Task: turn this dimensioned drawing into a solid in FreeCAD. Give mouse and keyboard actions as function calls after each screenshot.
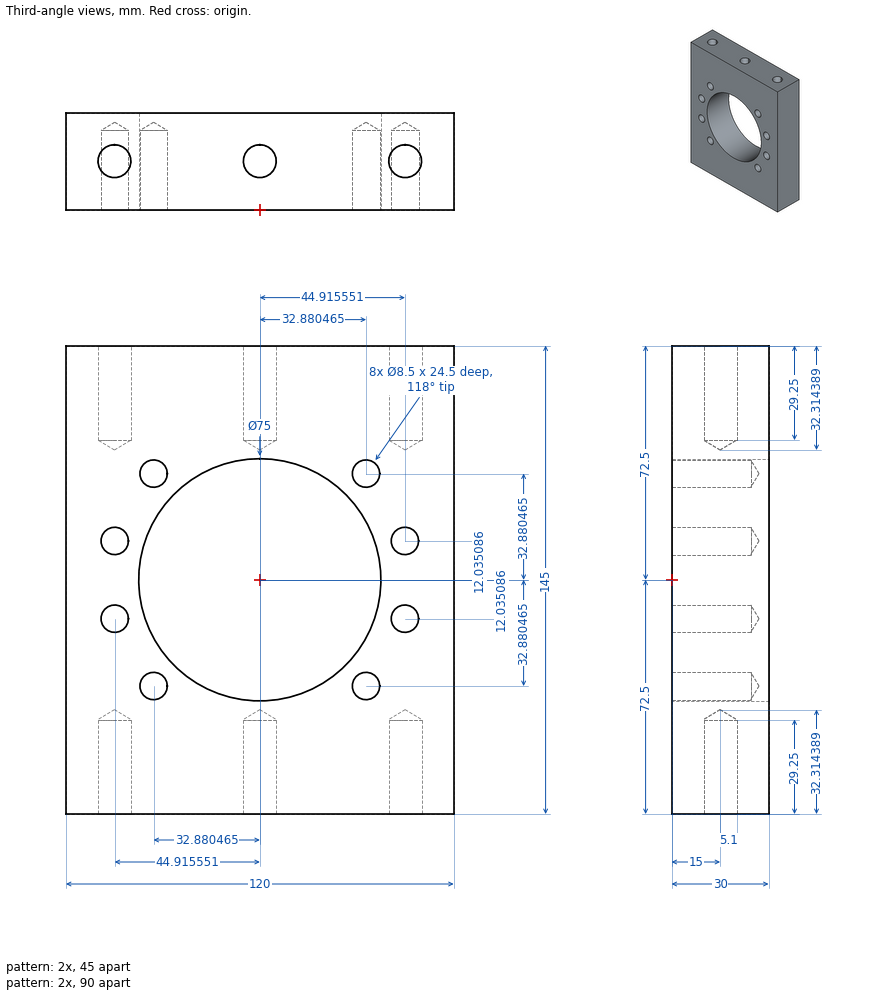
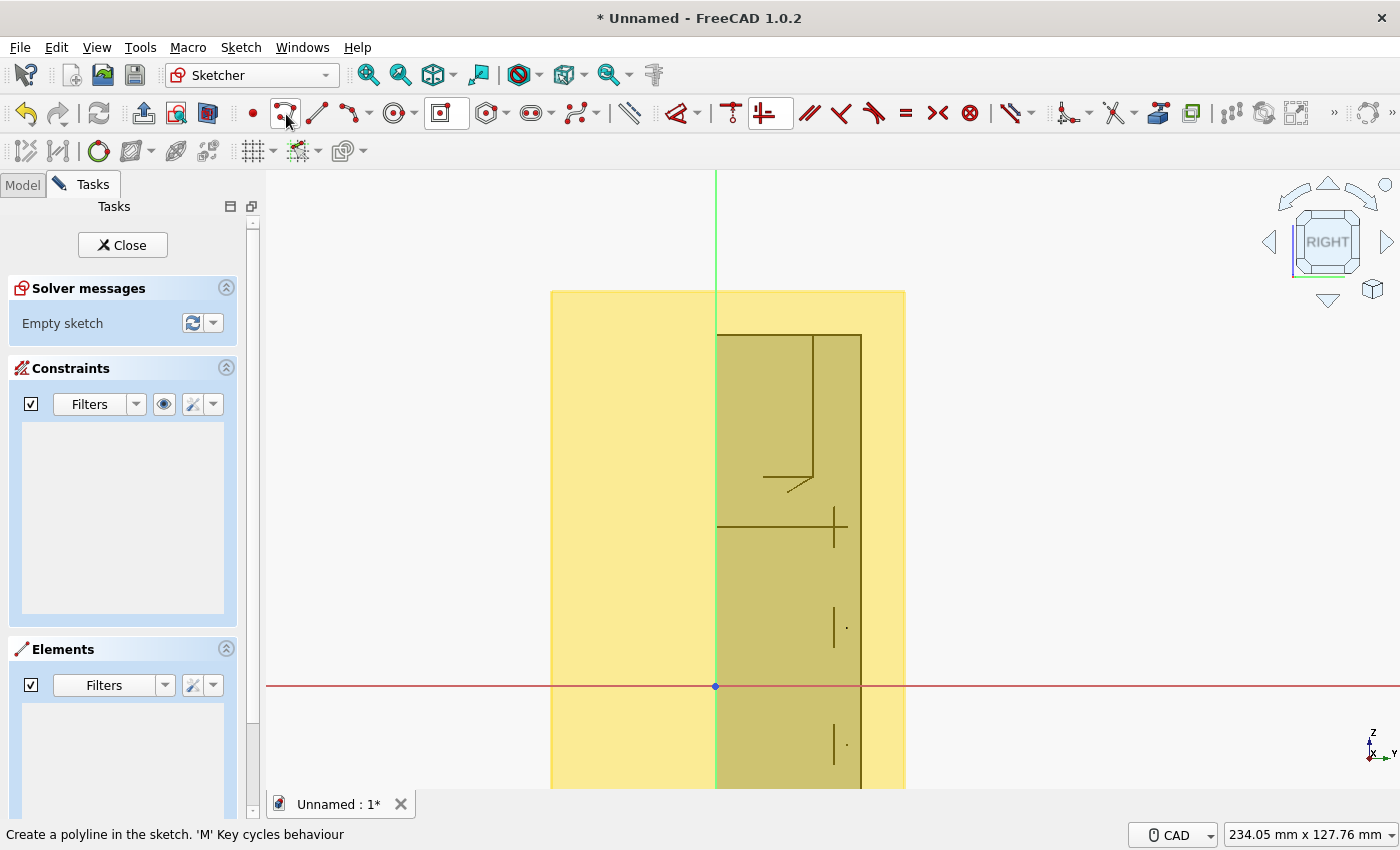
click(788, 492)
click(813, 477)
click(813, 335)
click(788, 335)
click(788, 493)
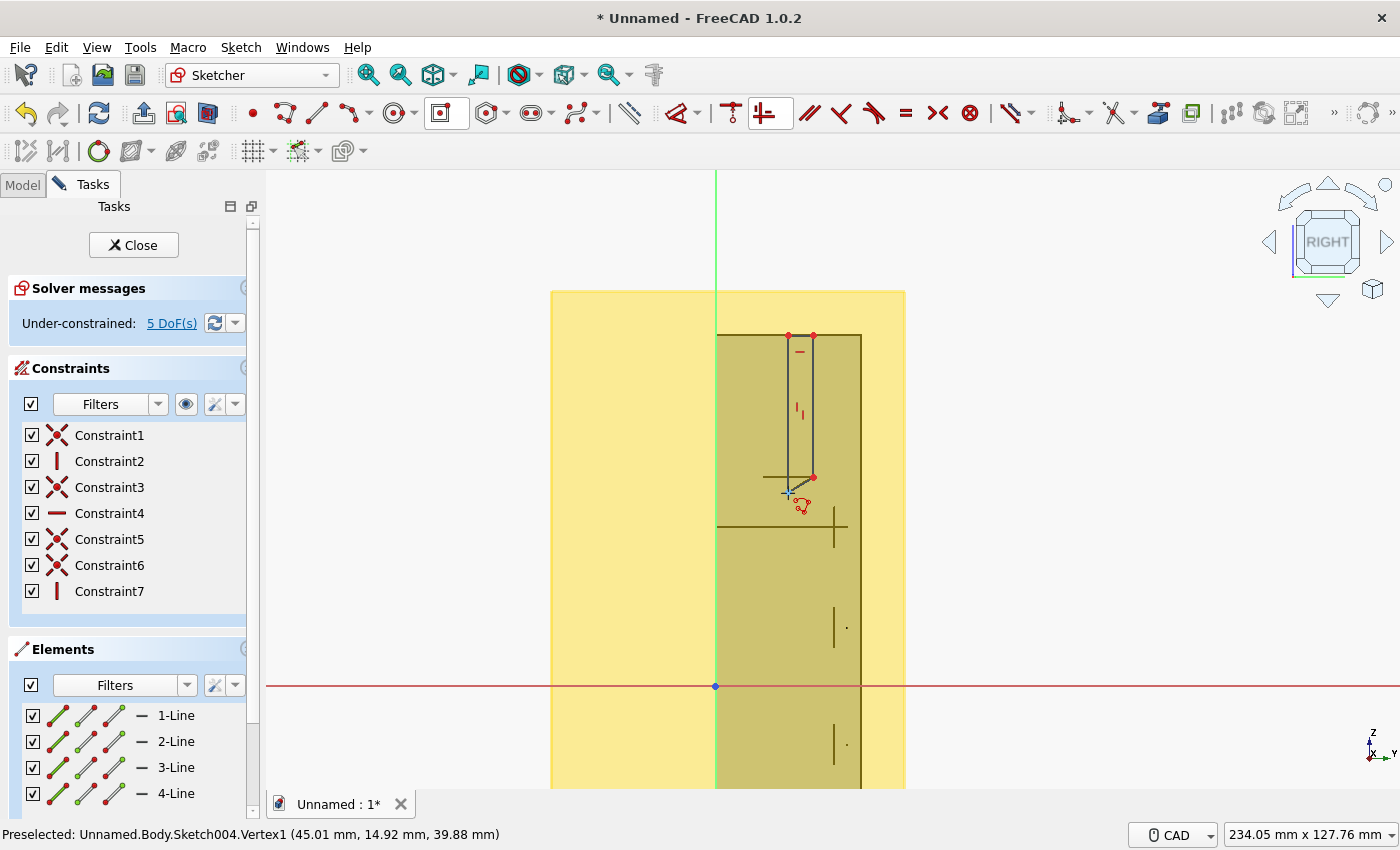
click(318, 114)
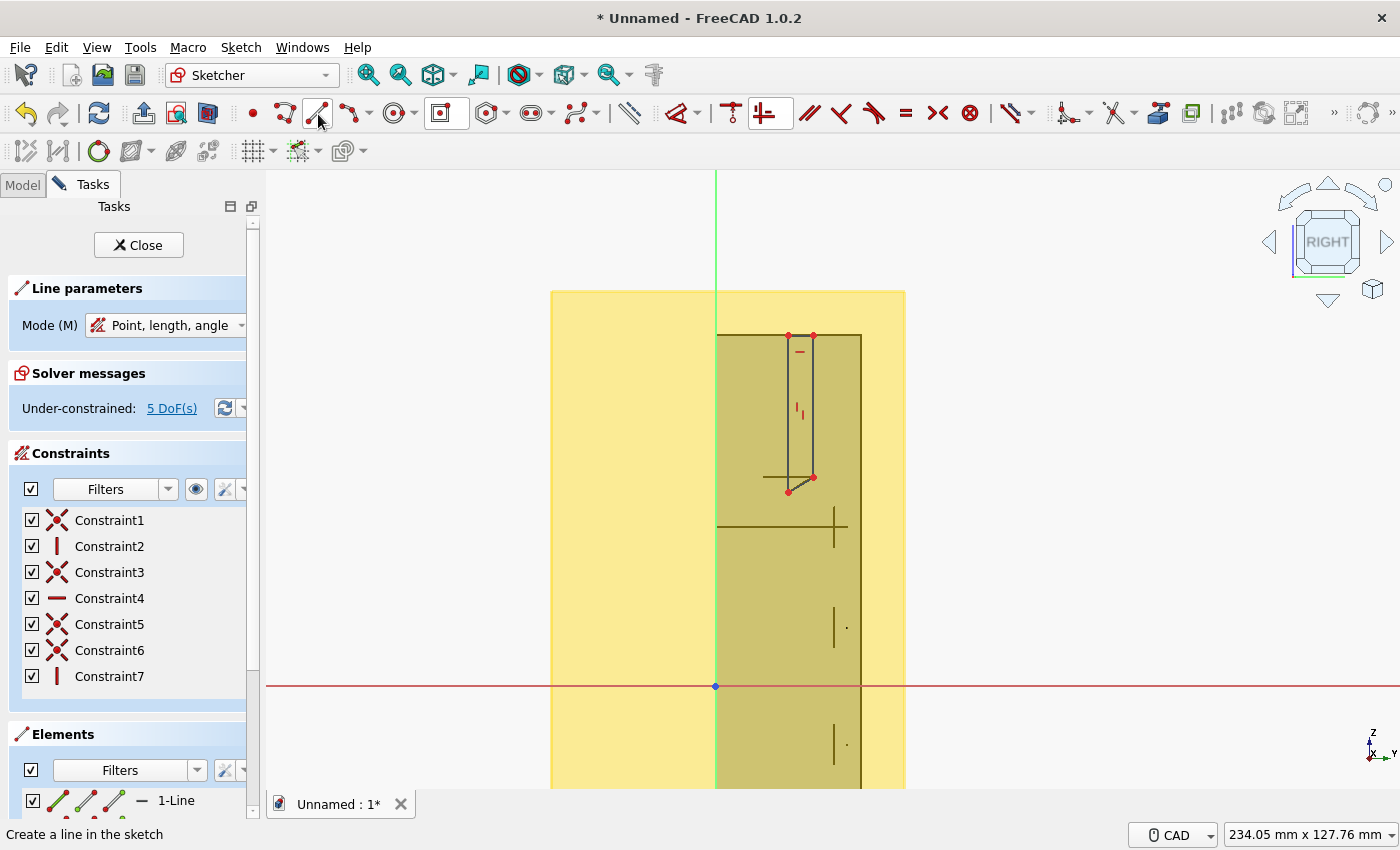
click(788, 319)
click(788, 272)
key(Escape)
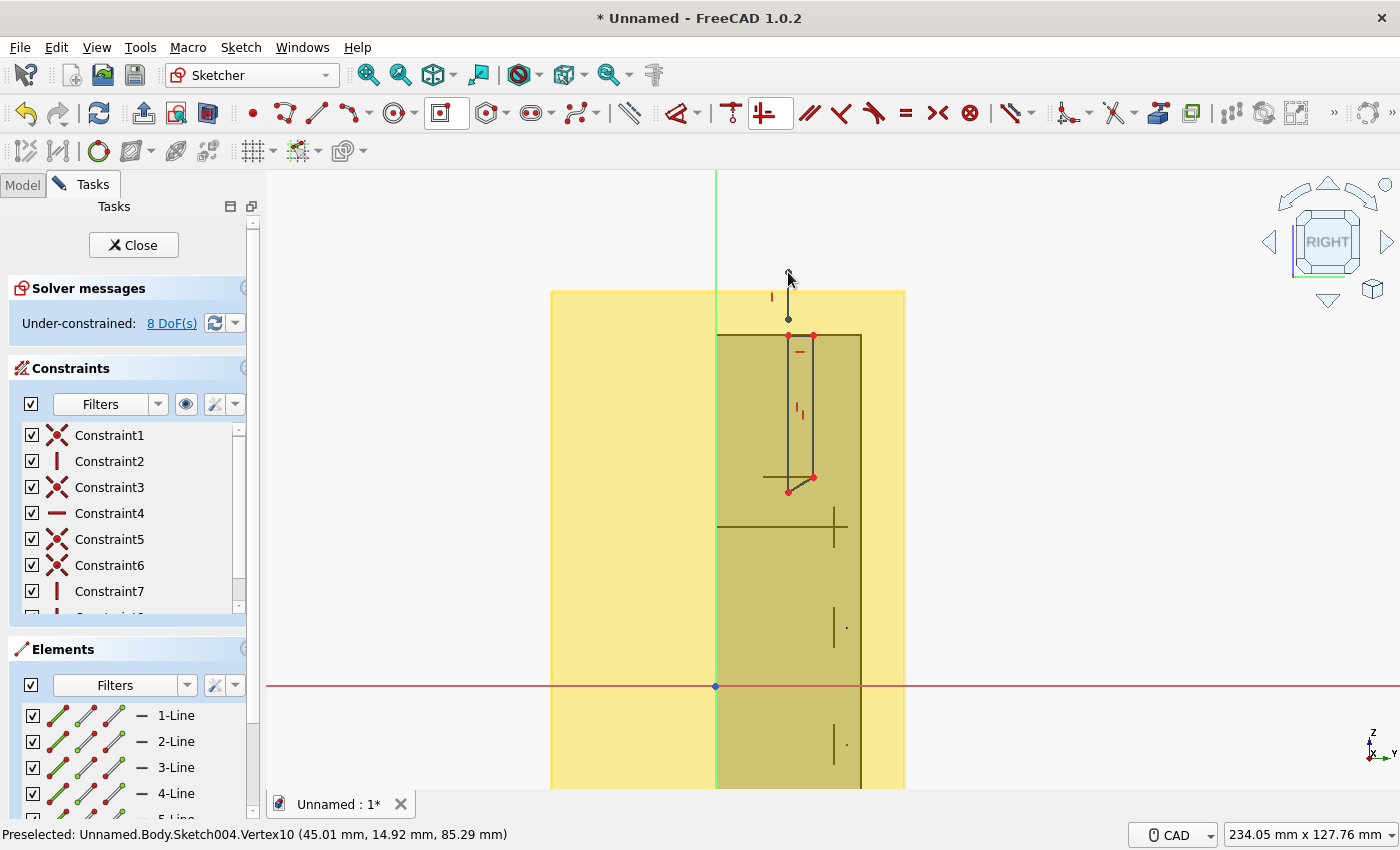
click(788, 306)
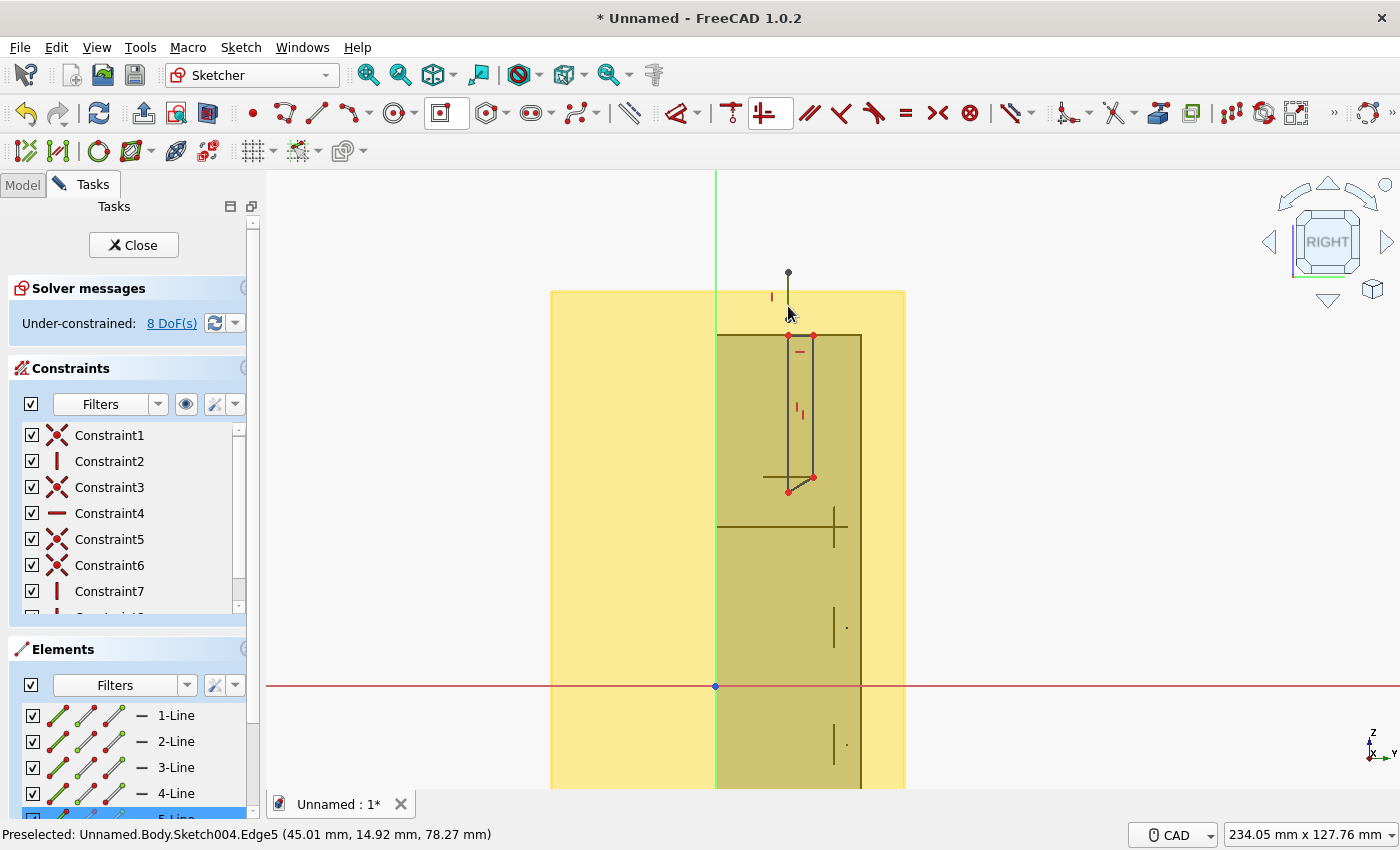
click(630, 114)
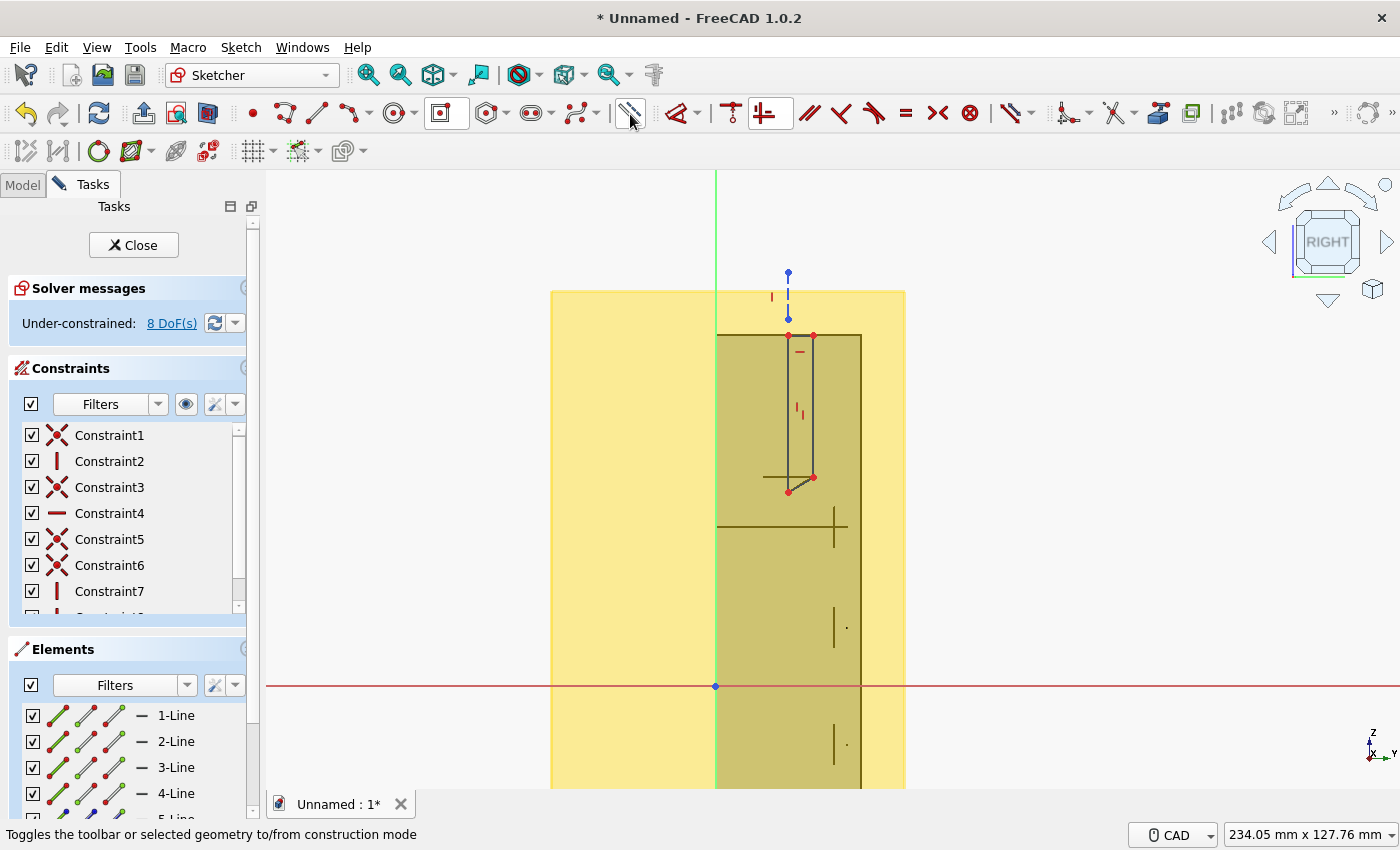
click(676, 114)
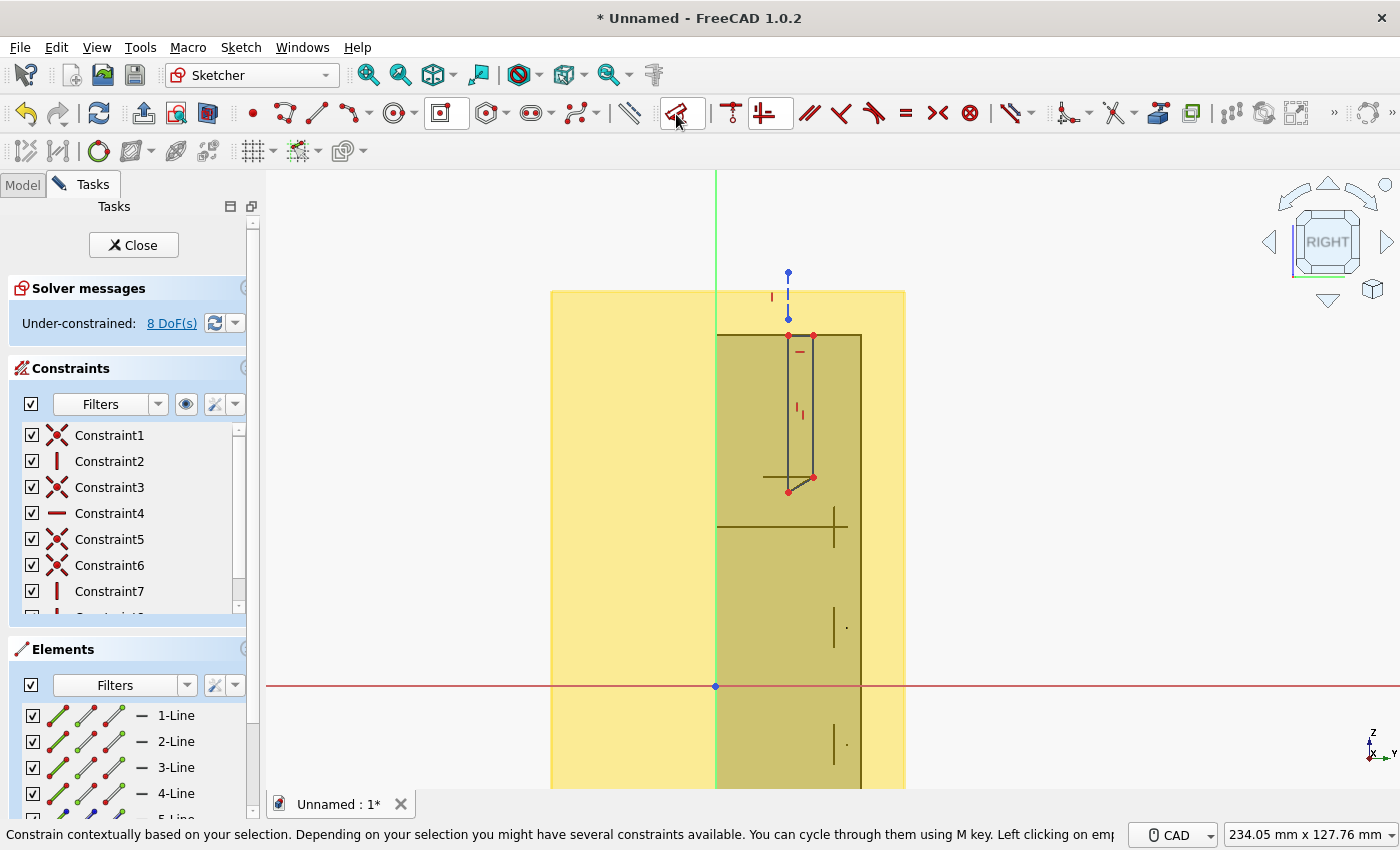
scroll(803, 336, up, 3)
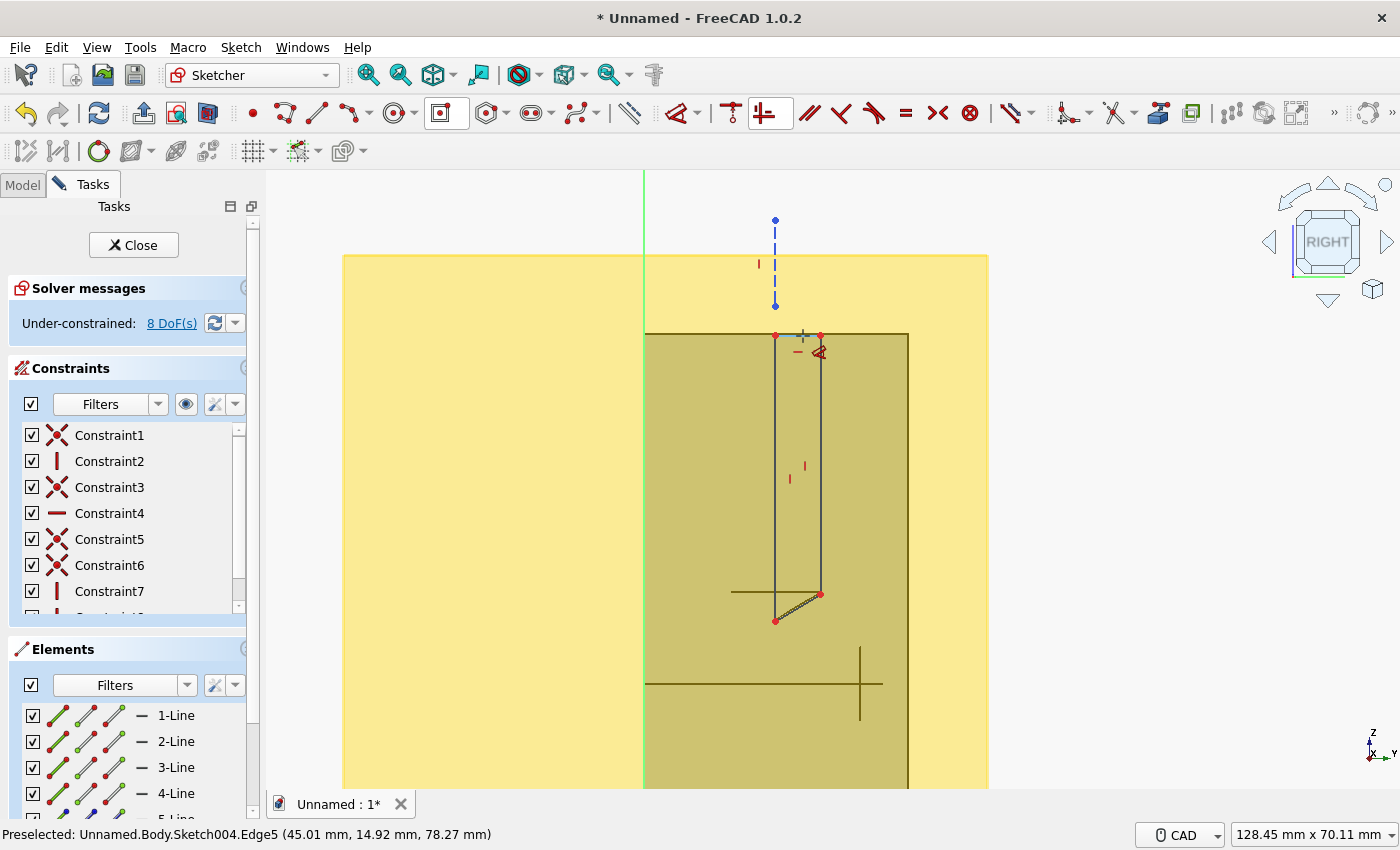
click(803, 336)
click(798, 302)